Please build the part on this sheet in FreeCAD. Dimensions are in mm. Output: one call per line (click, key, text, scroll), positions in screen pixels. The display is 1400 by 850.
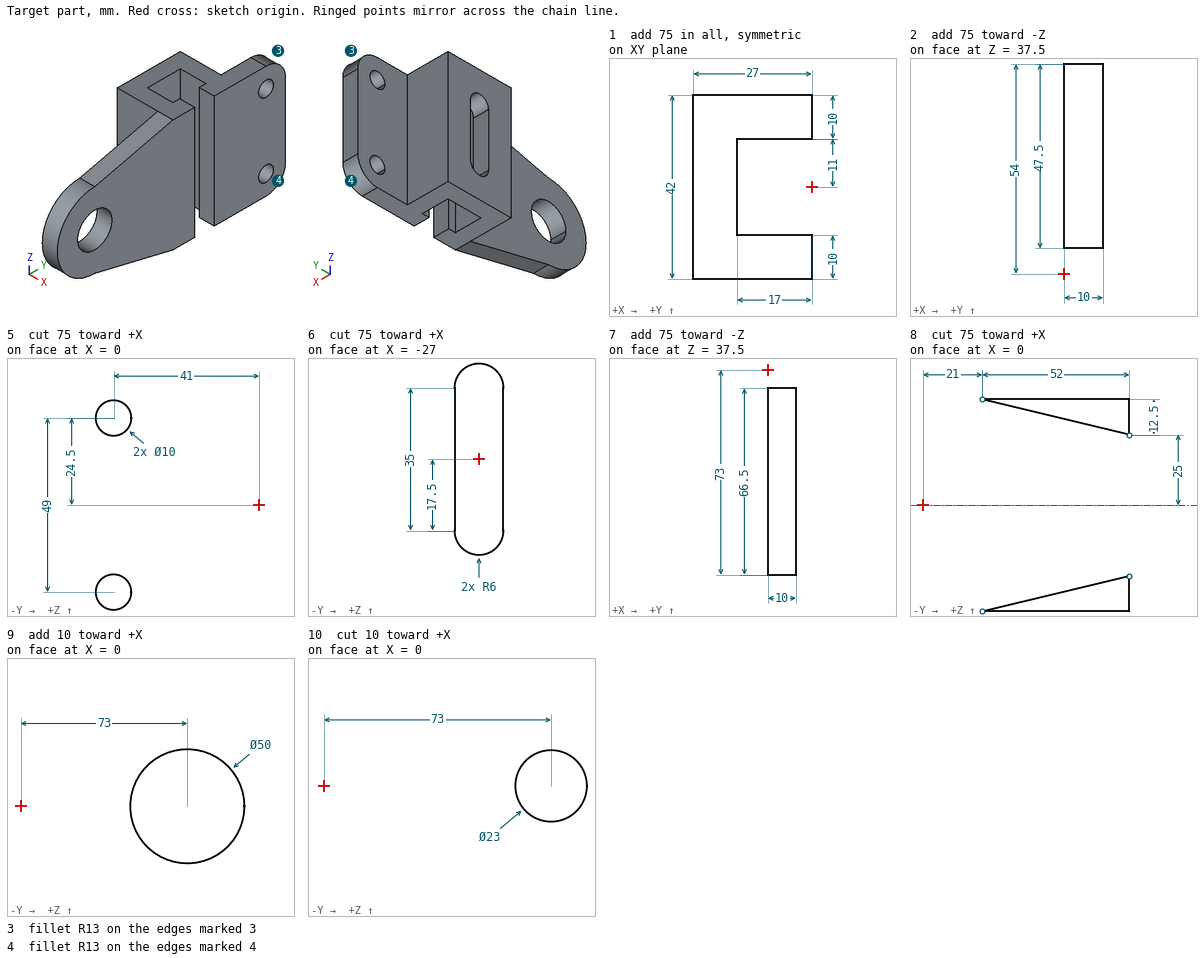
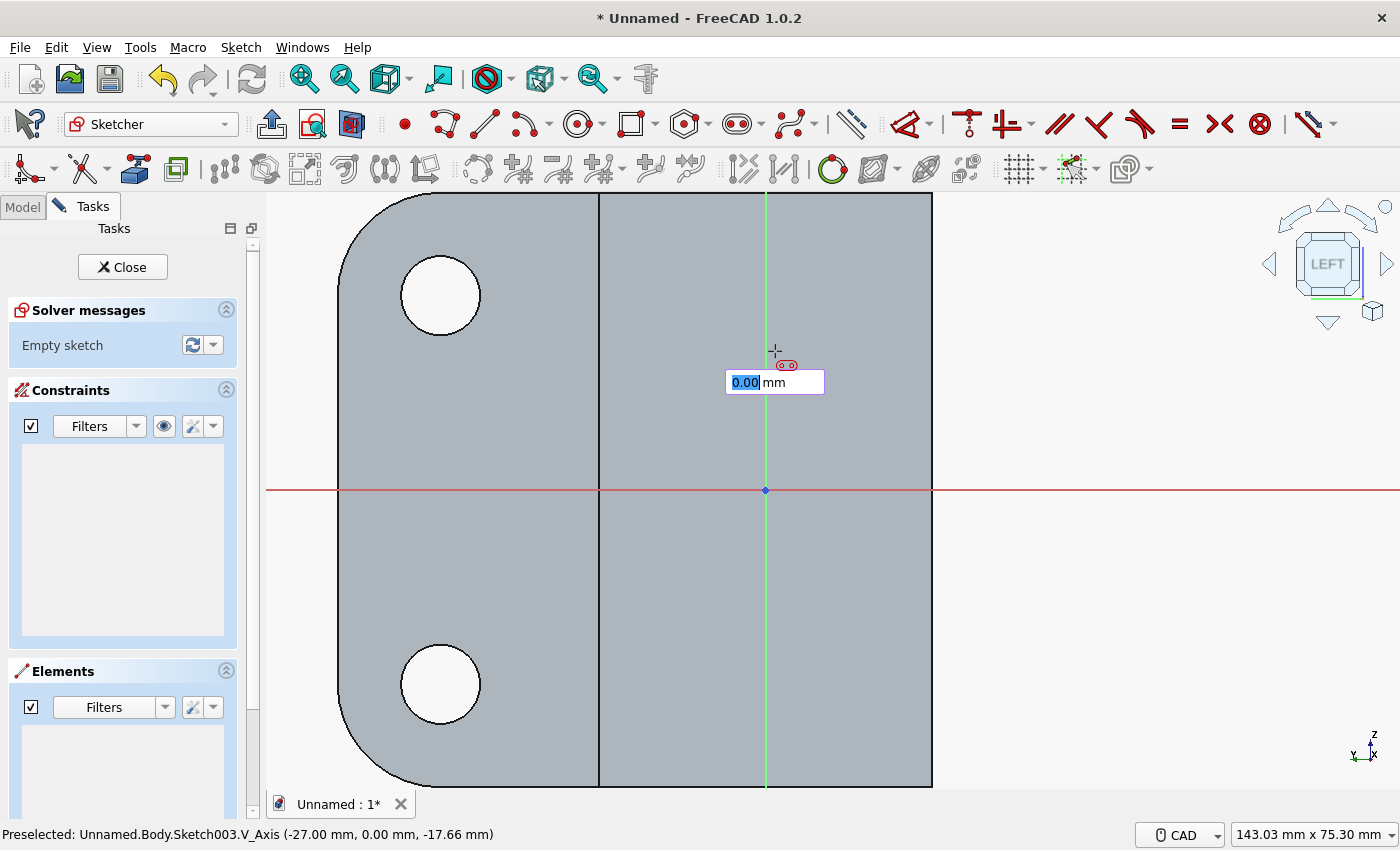
click(718, 448)
key(Escape)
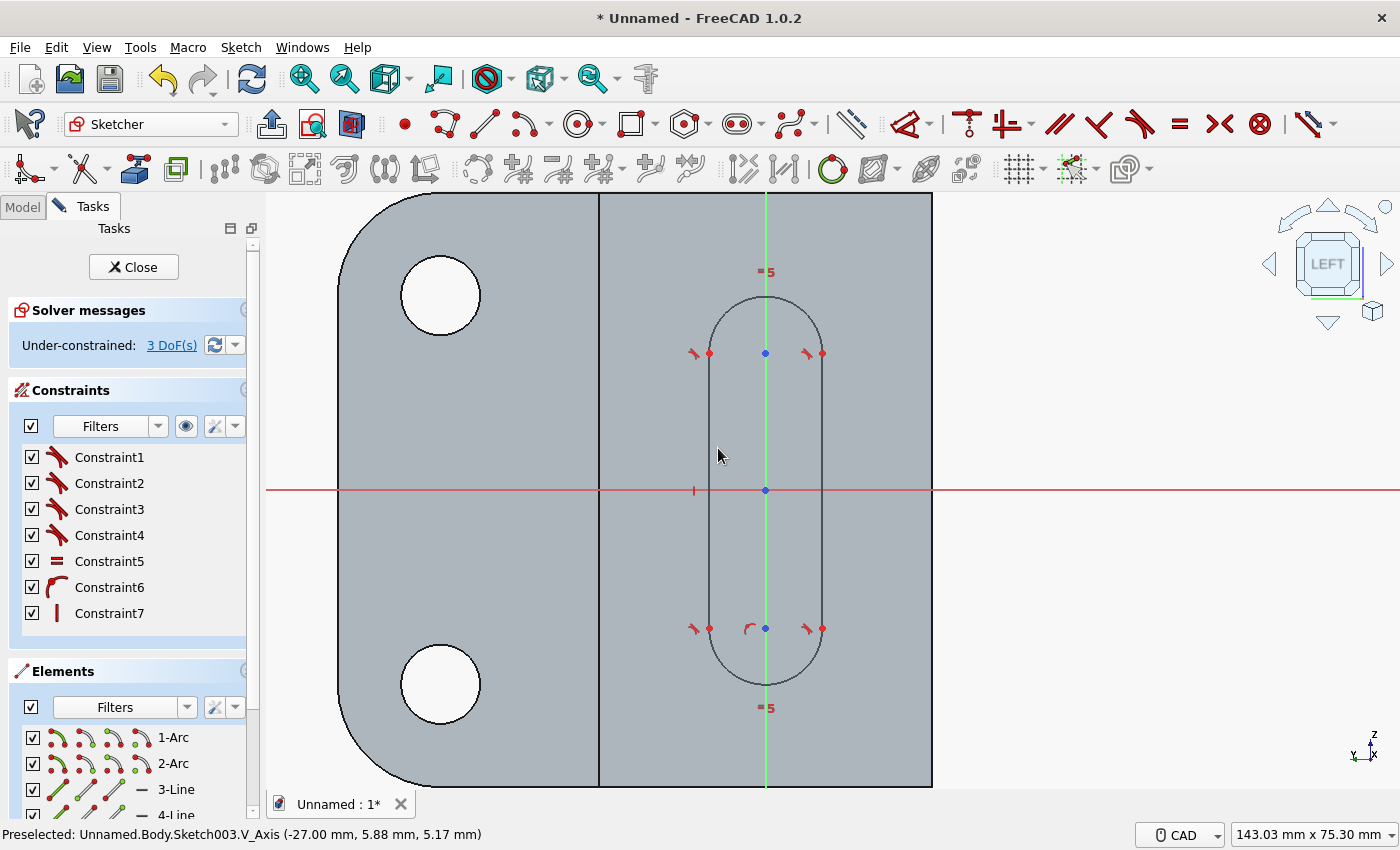
key(d)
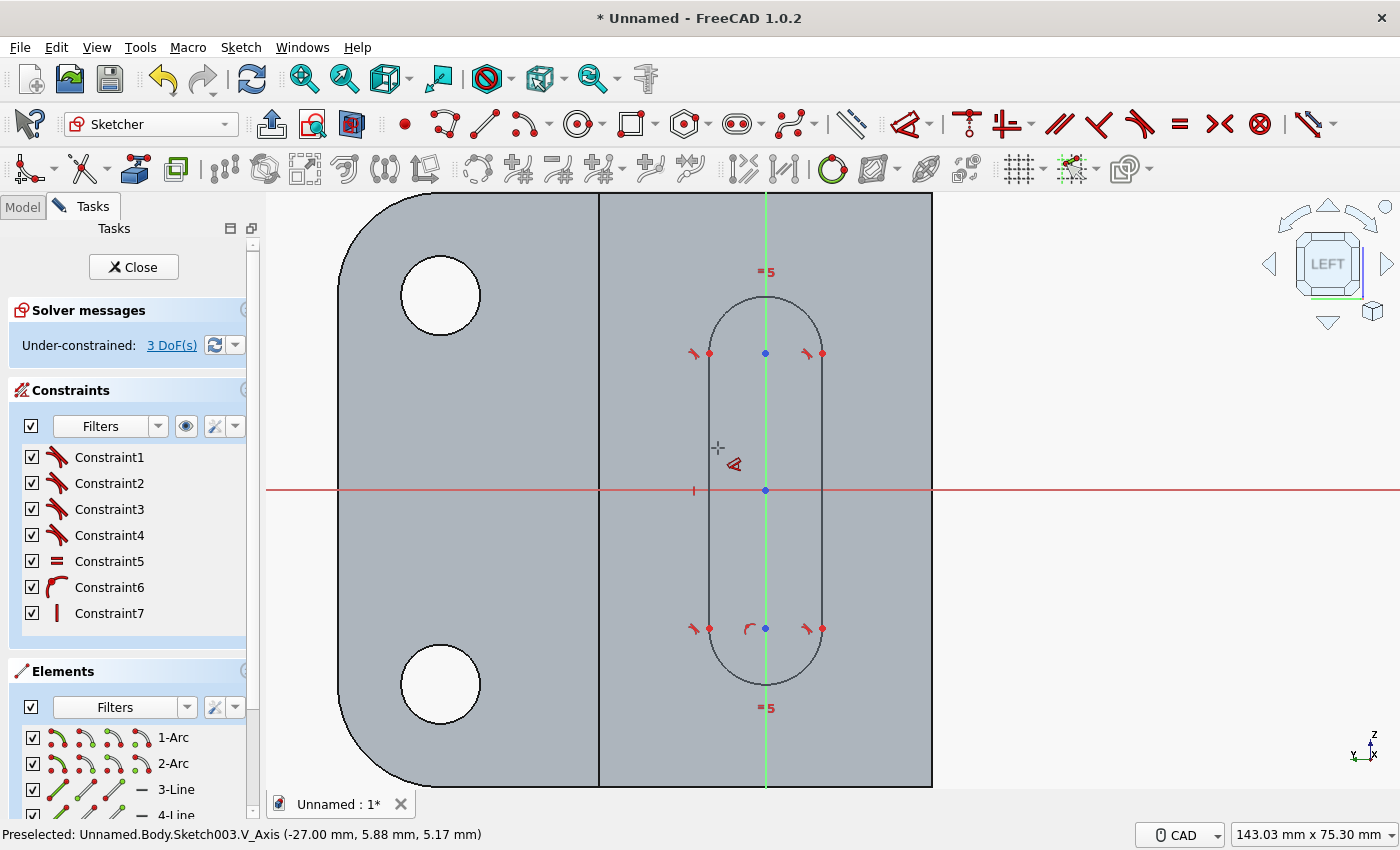
click(732, 674)
click(713, 700)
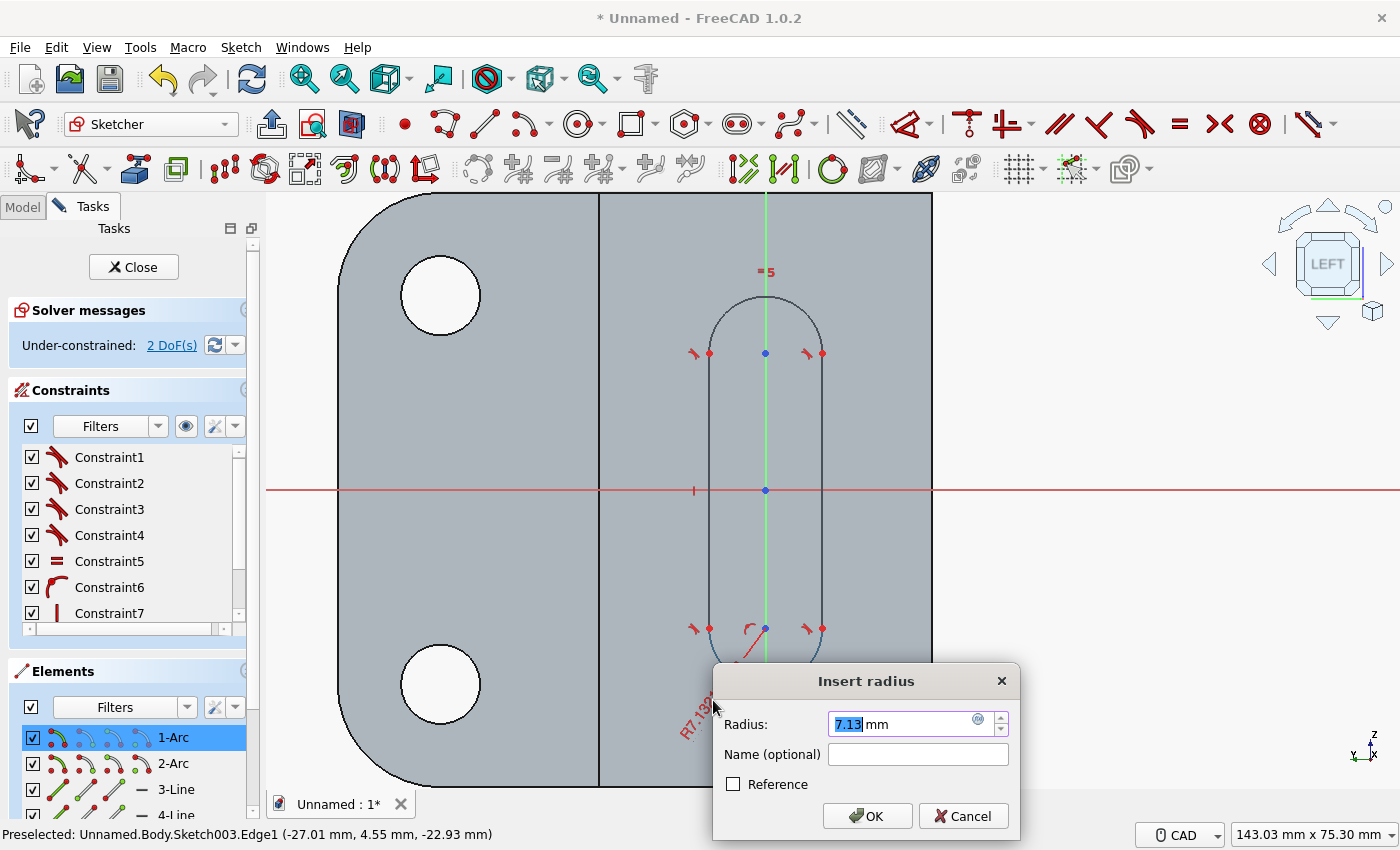
text(6)
key(Return)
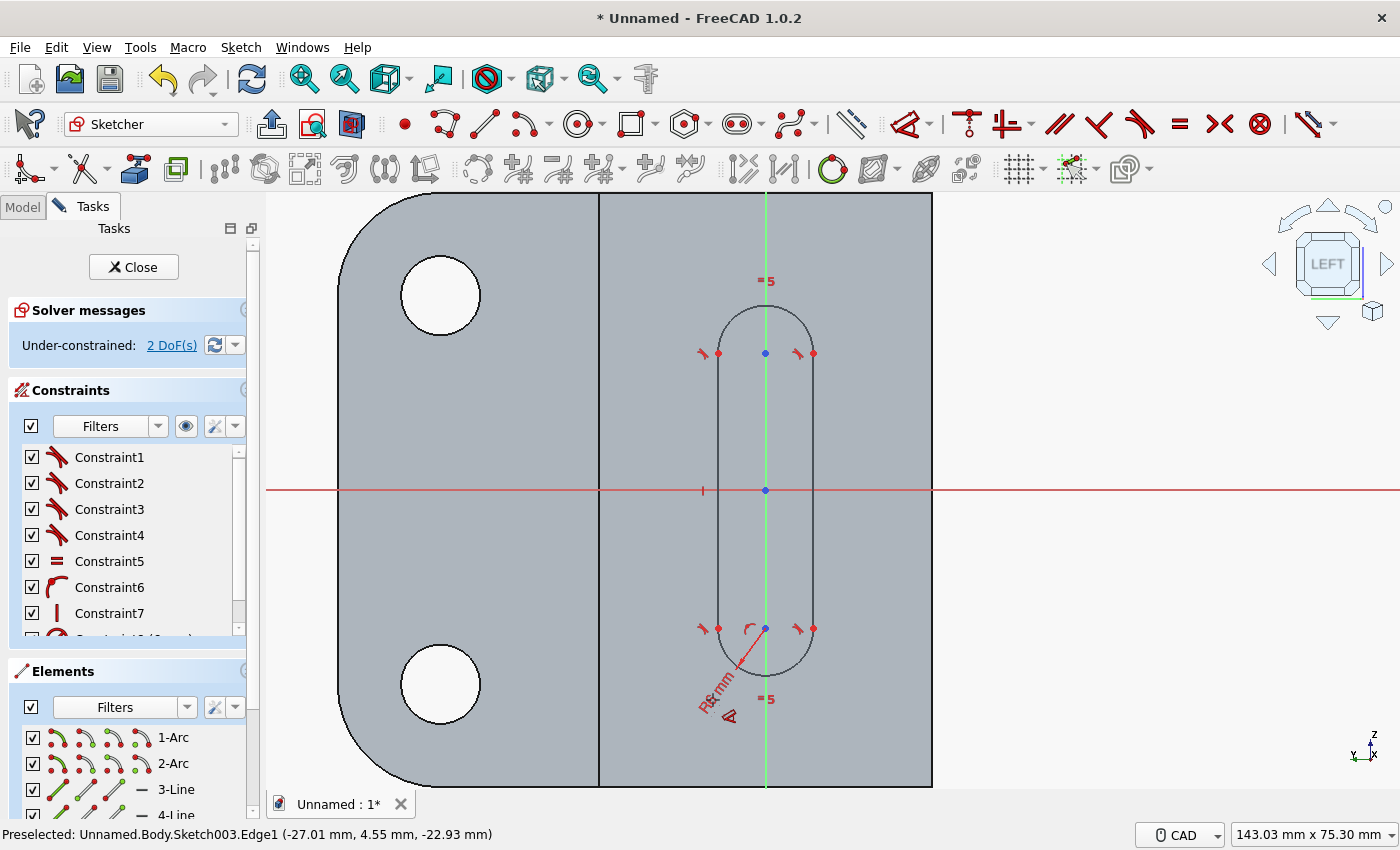
click(718, 546)
click(684, 427)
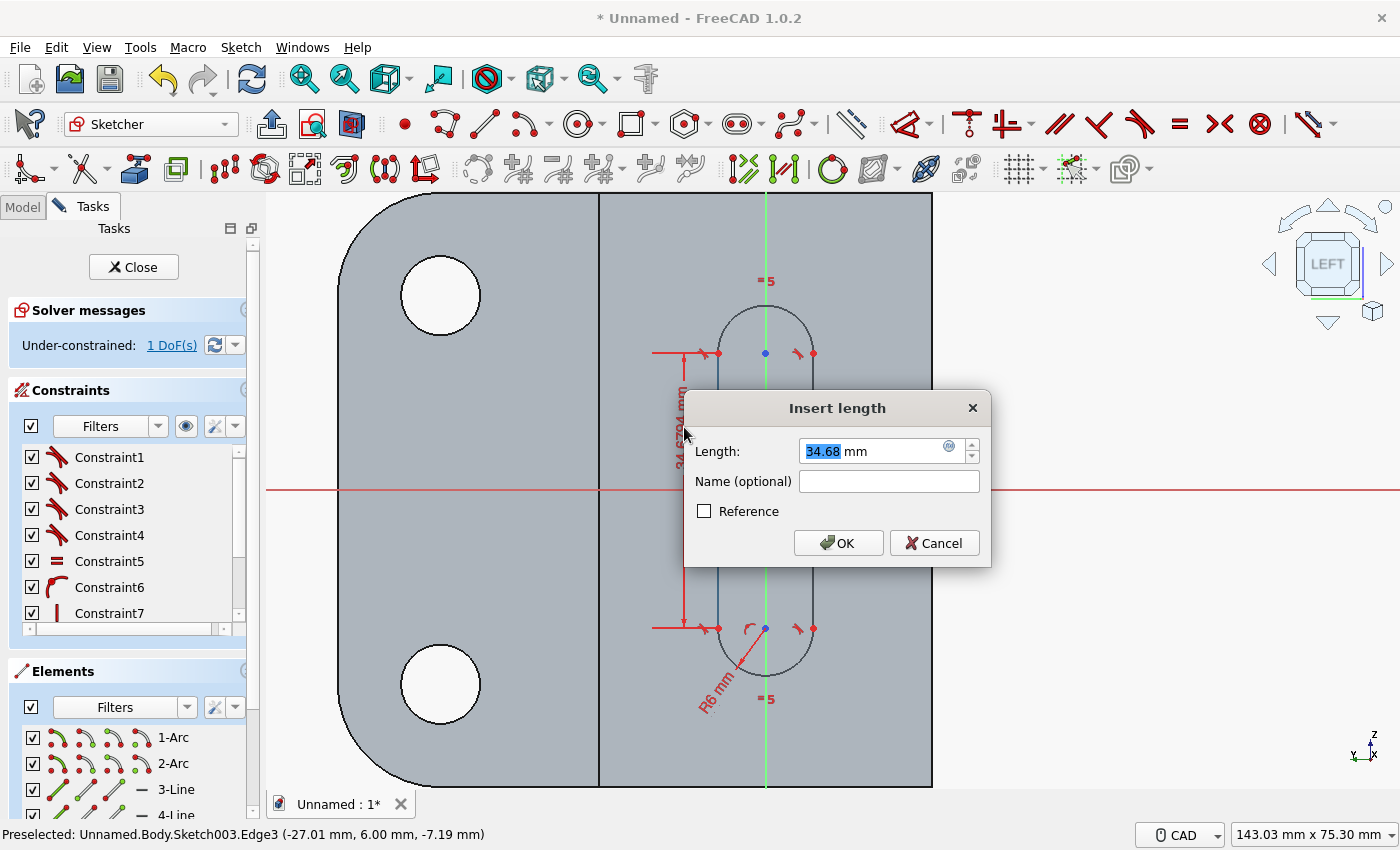
text(35)
key(Return)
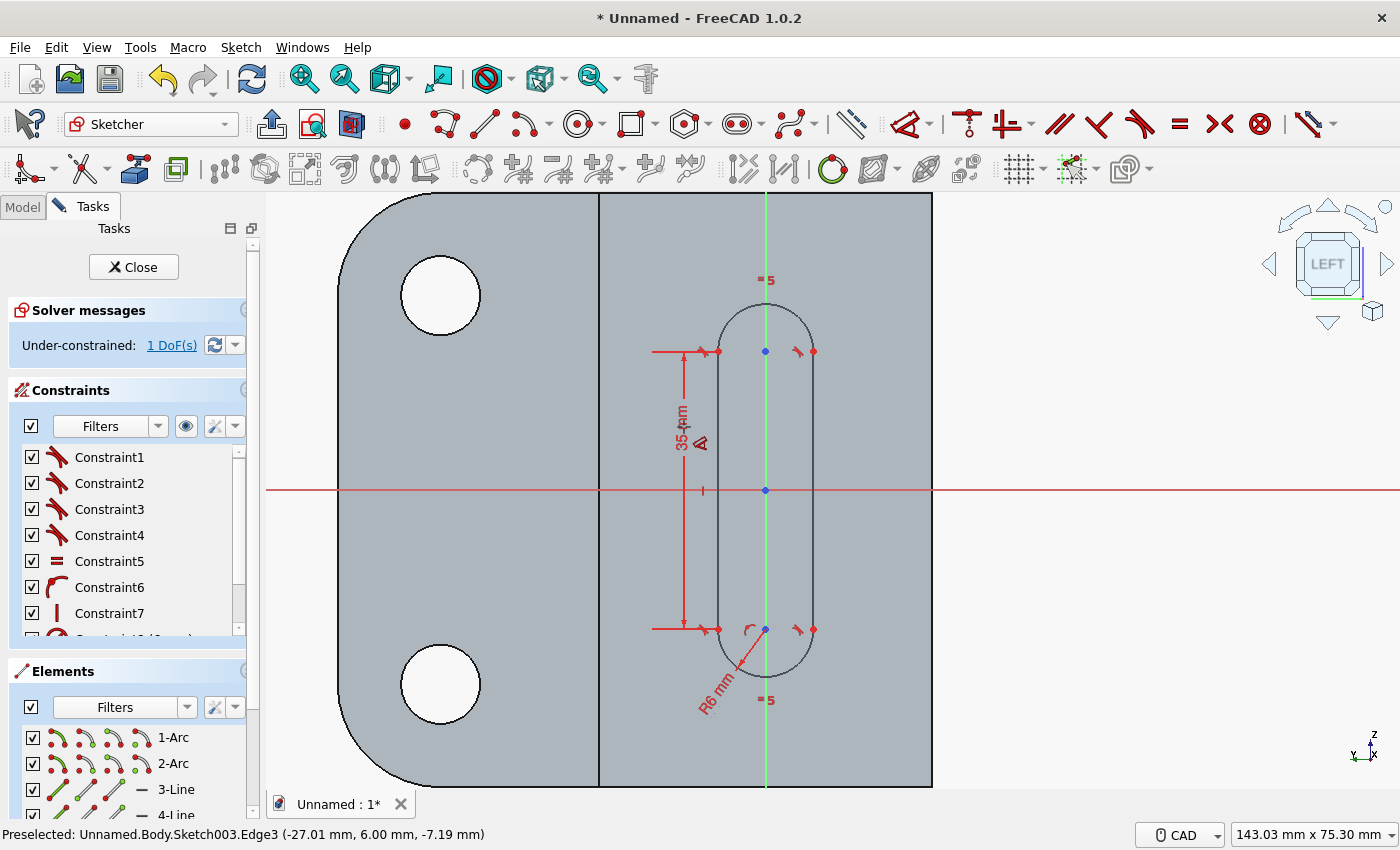
click(718, 629)
click(684, 560)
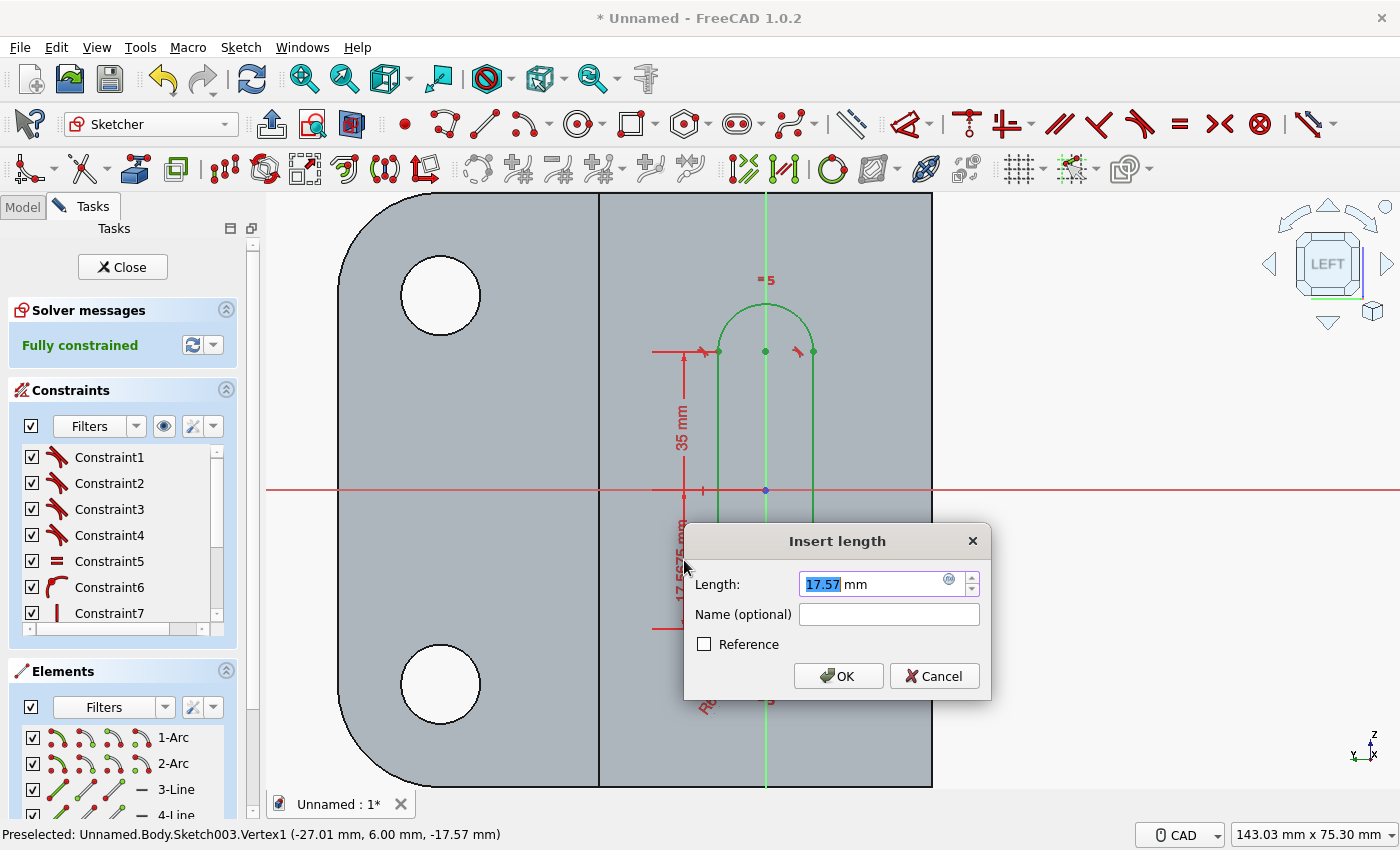
text(17.5)
key(Return)
key(Escape)